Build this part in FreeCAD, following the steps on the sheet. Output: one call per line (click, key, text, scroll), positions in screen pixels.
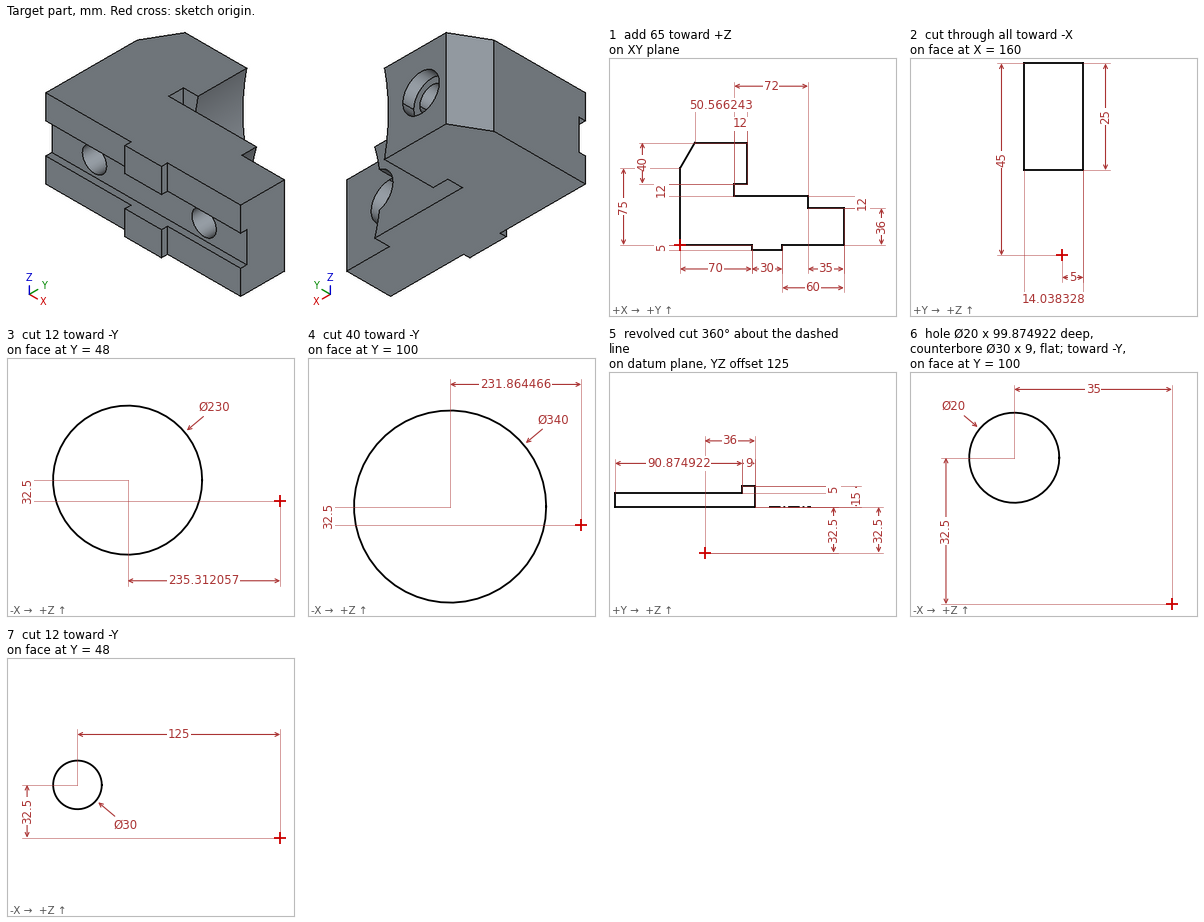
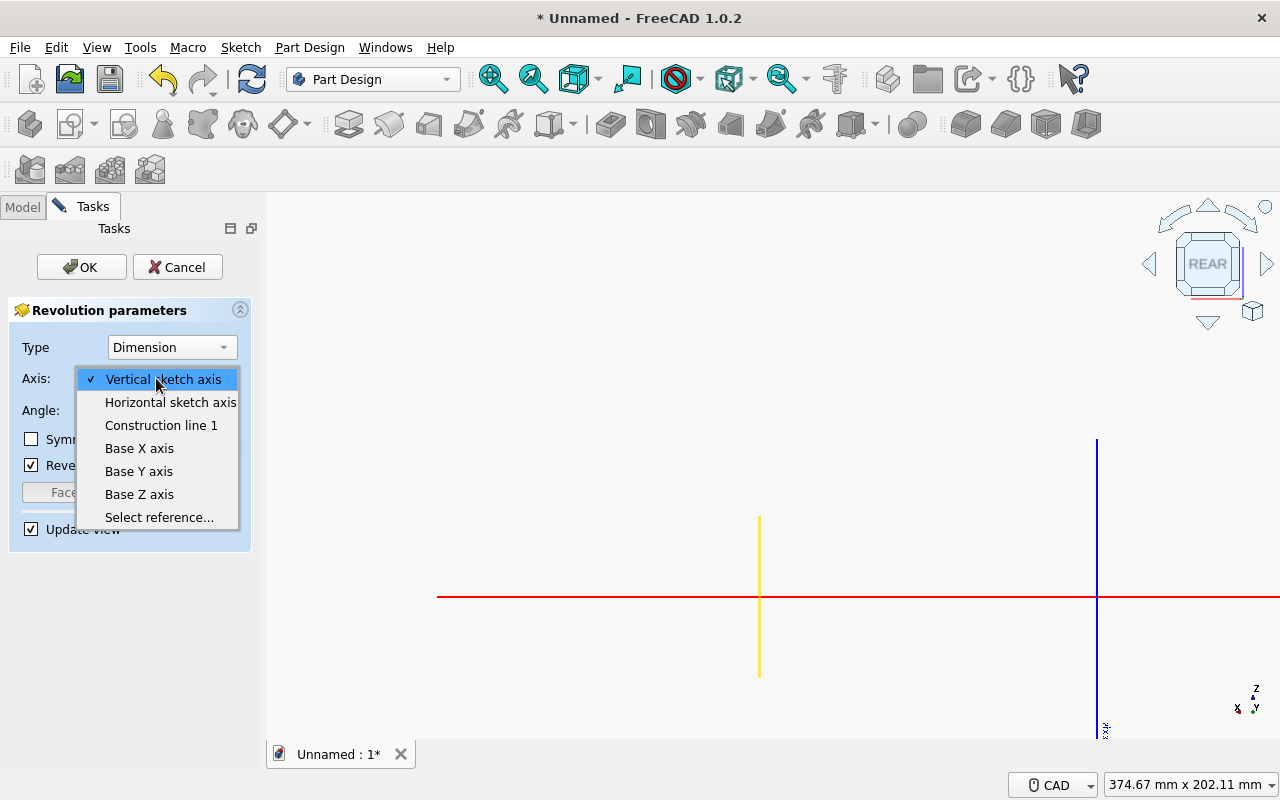
click(156, 426)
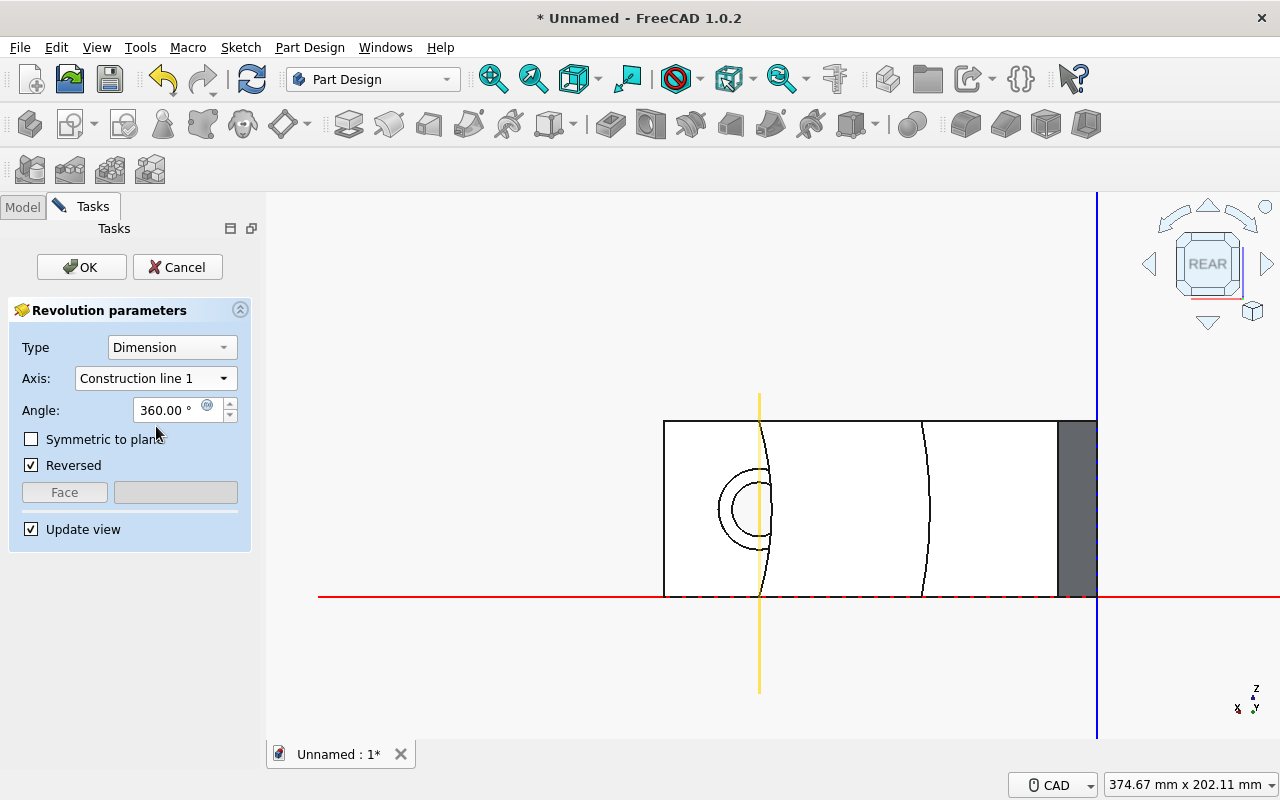
click(82, 267)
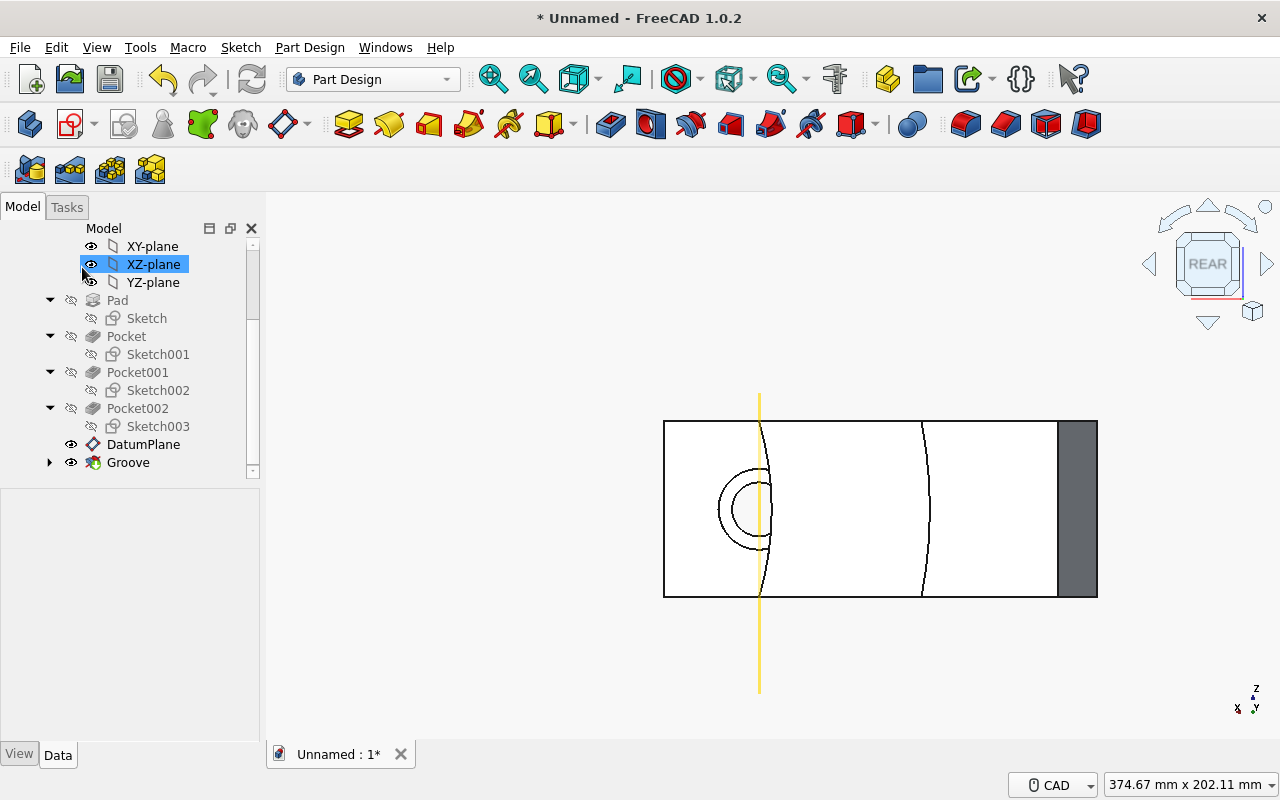
click(116, 444)
key(space)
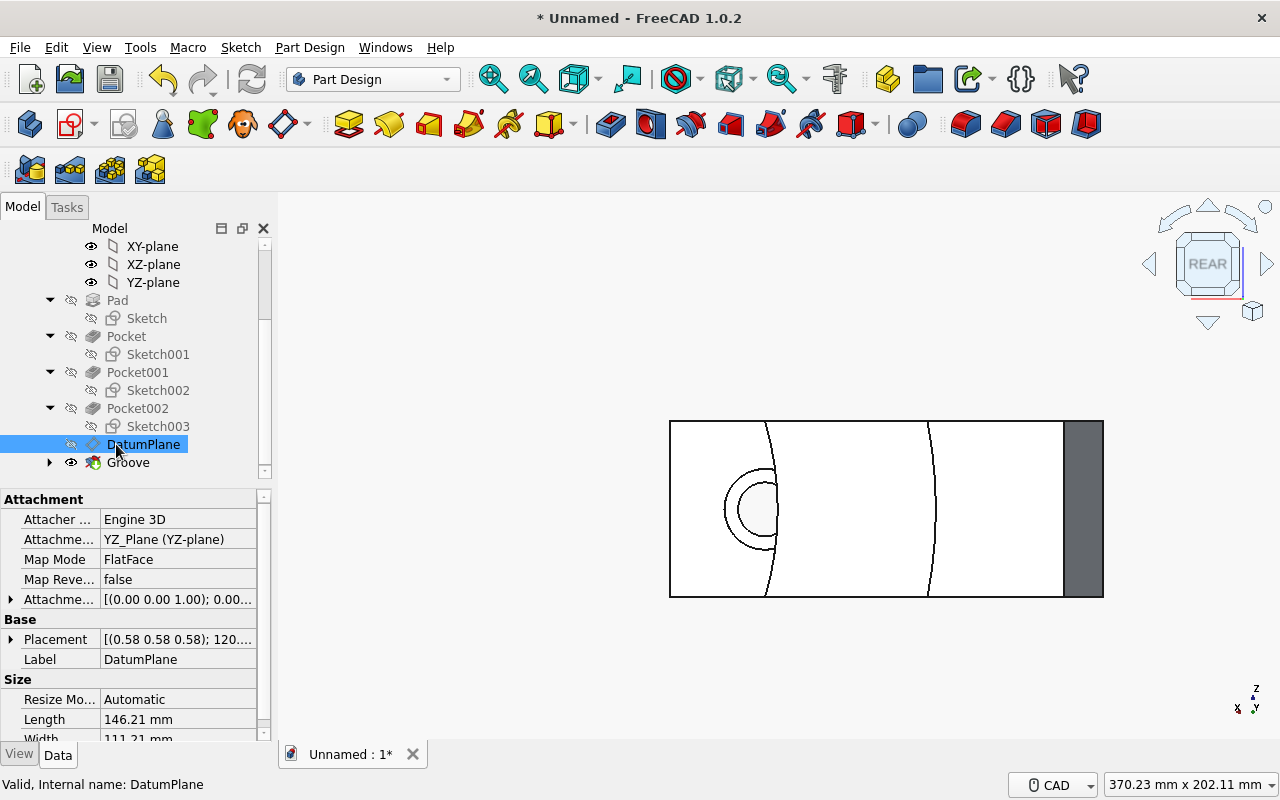
key(v)
key(f)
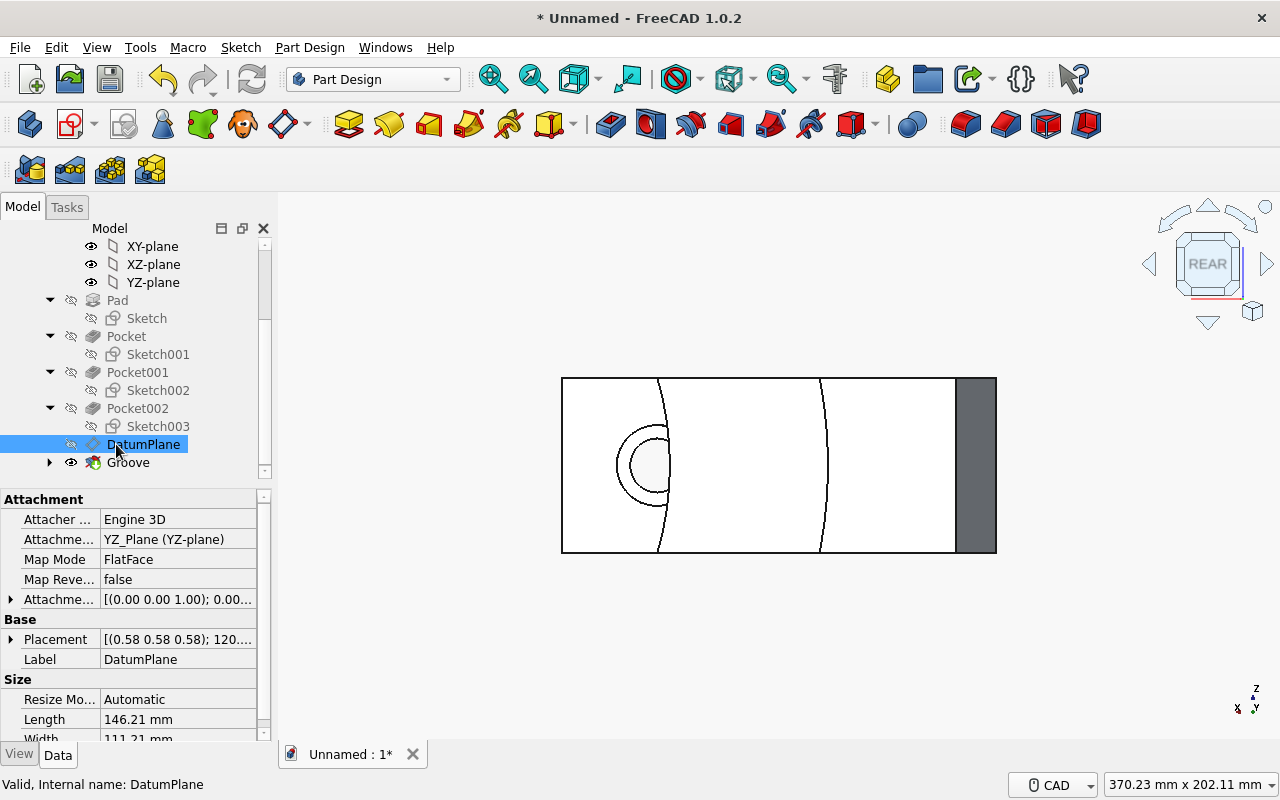
click(888, 439)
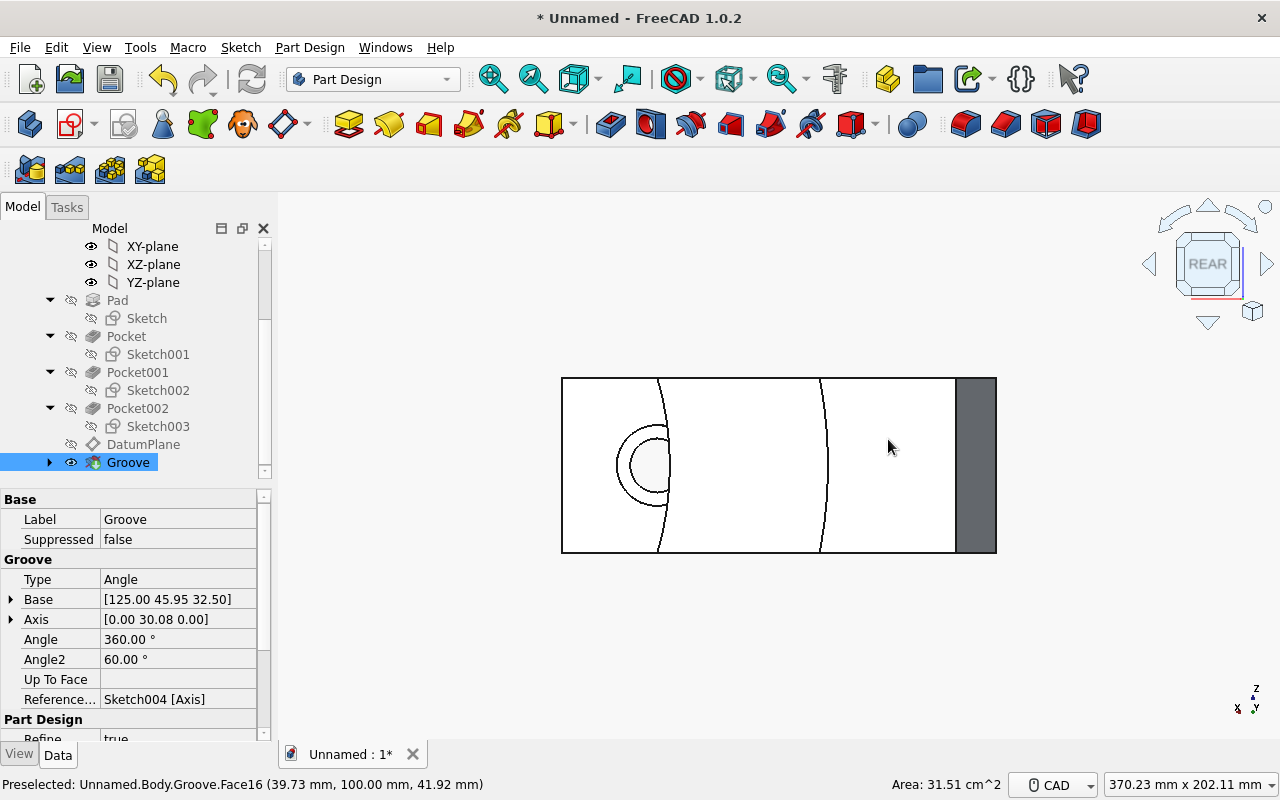
click(70, 124)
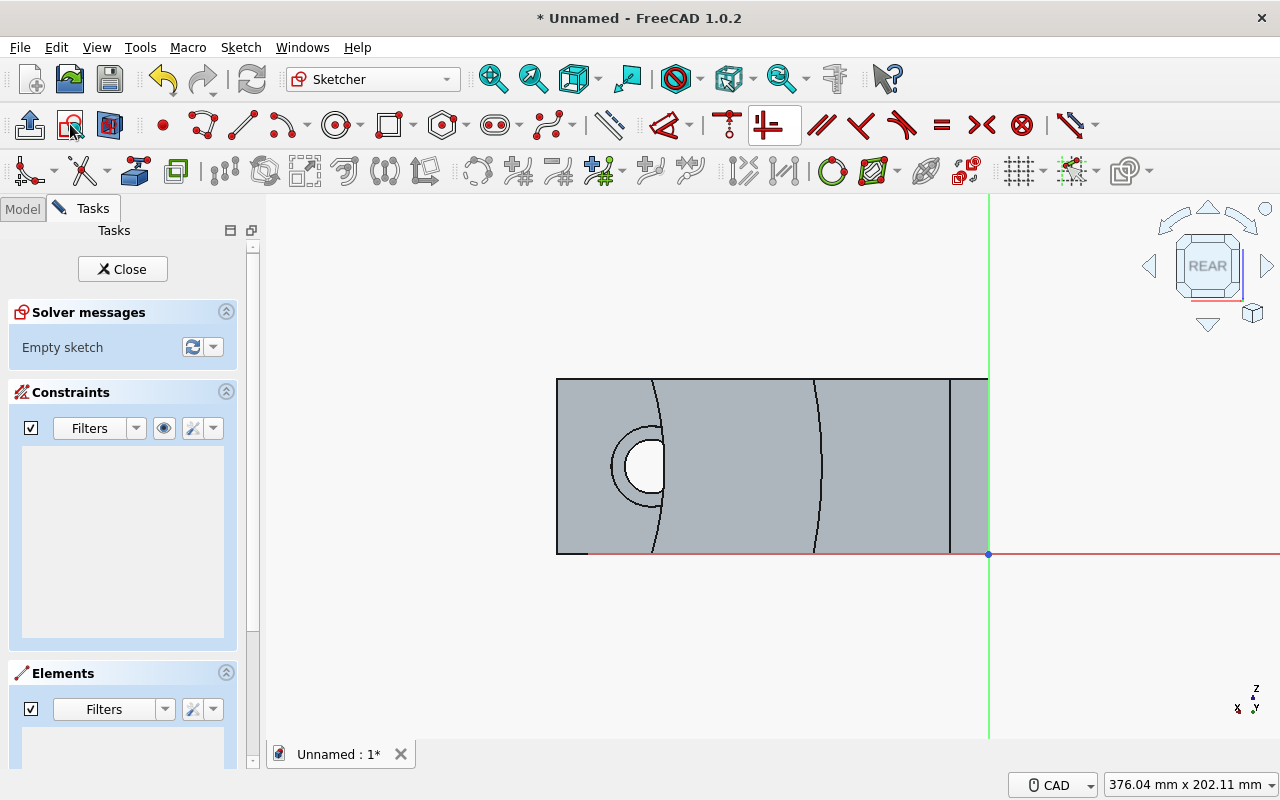
scroll(1024, 510, up, 6)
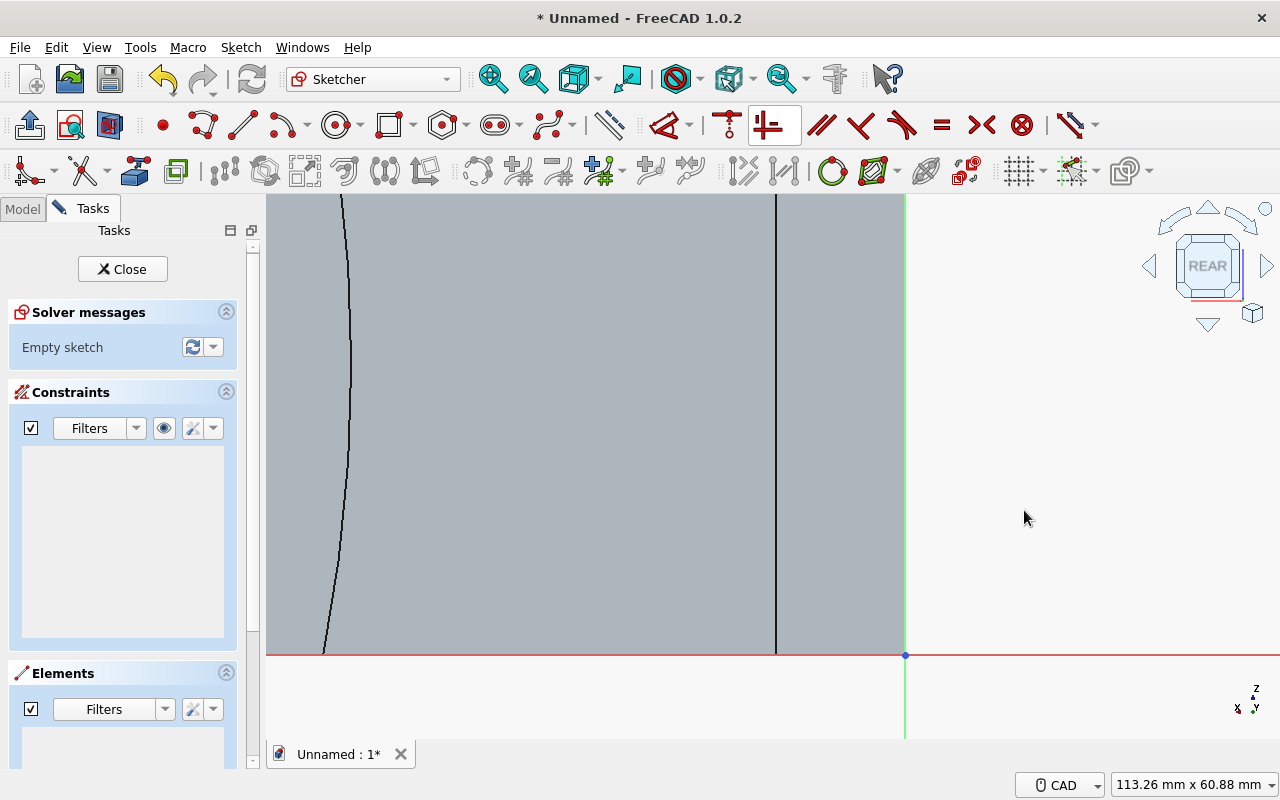
key(g)
key(c)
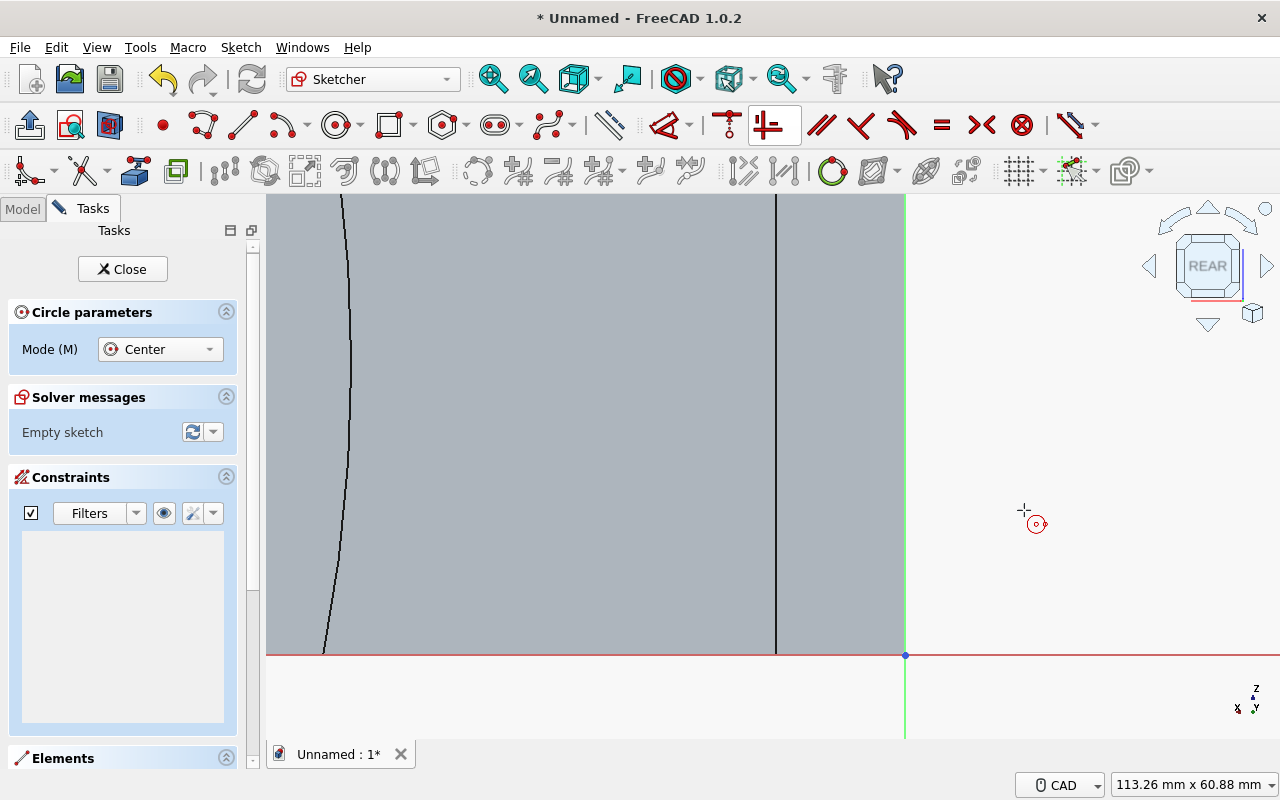
click(592, 364)
move(655, 301)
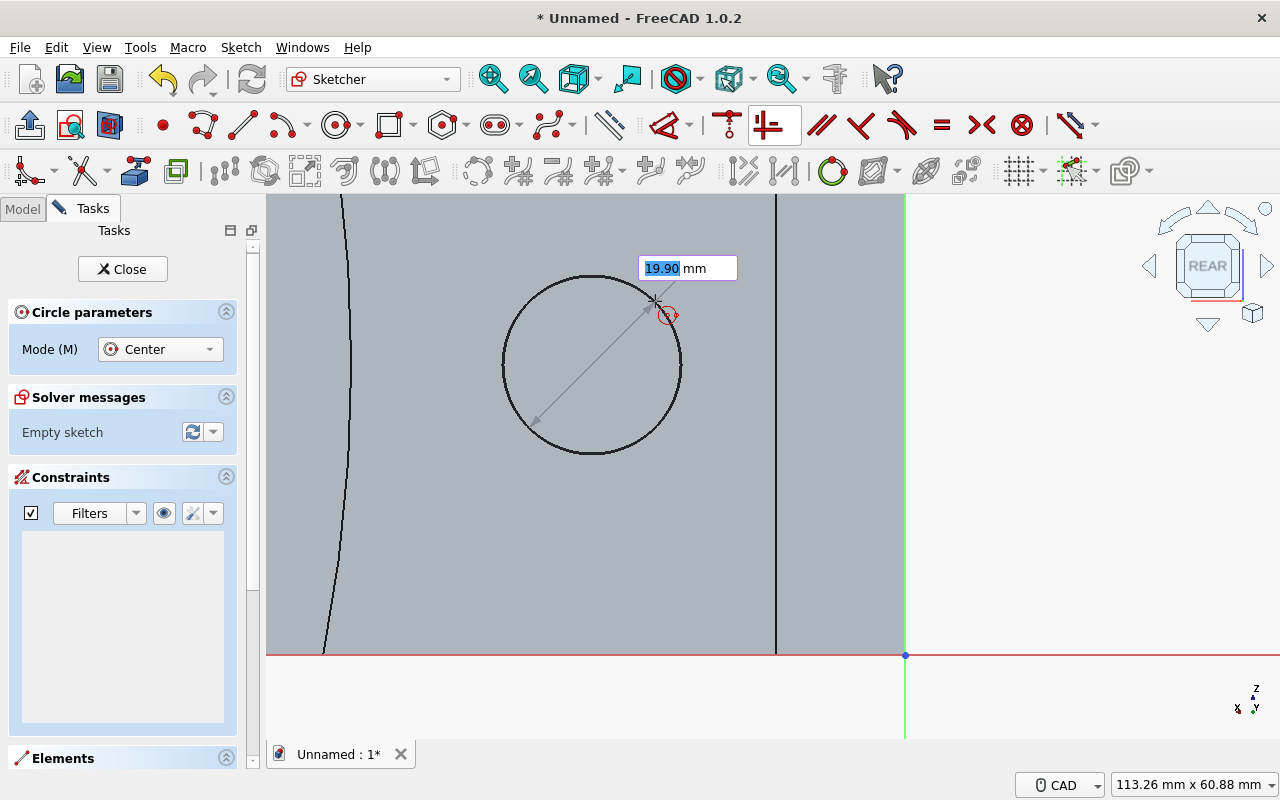
text(20)
key(Return)
key(Escape)